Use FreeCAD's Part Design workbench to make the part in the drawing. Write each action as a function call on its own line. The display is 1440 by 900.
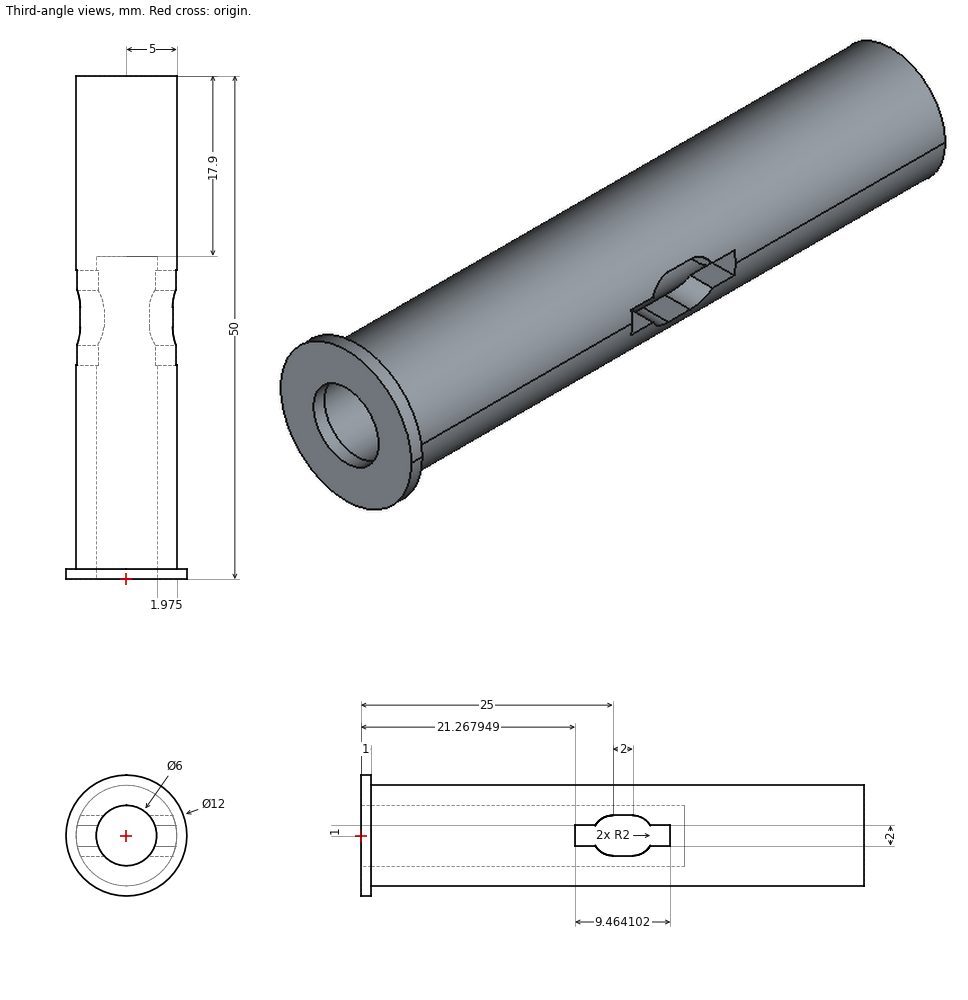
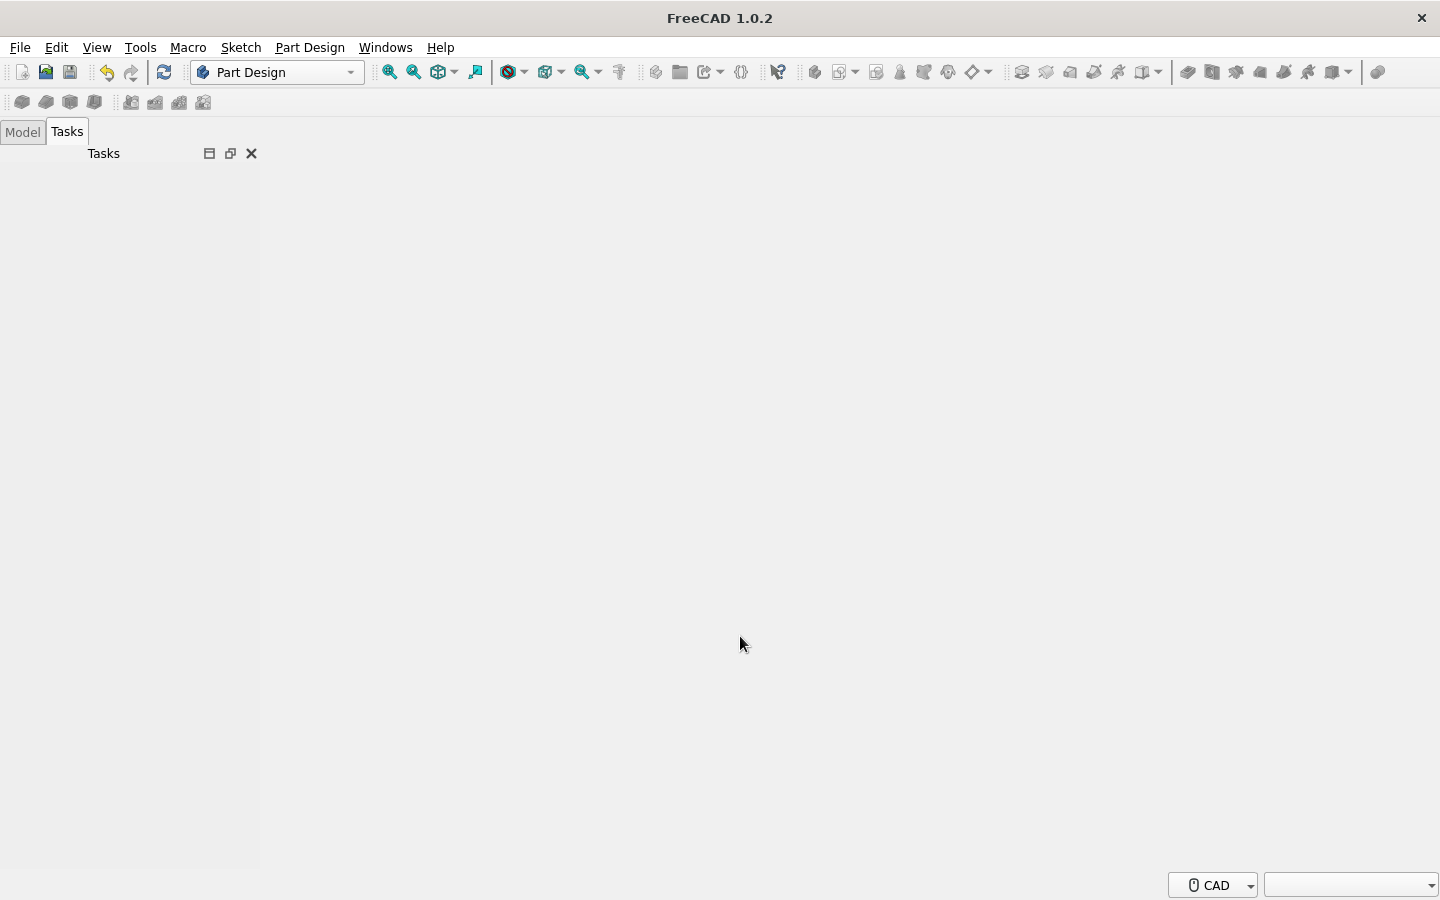
key(ctrl+n)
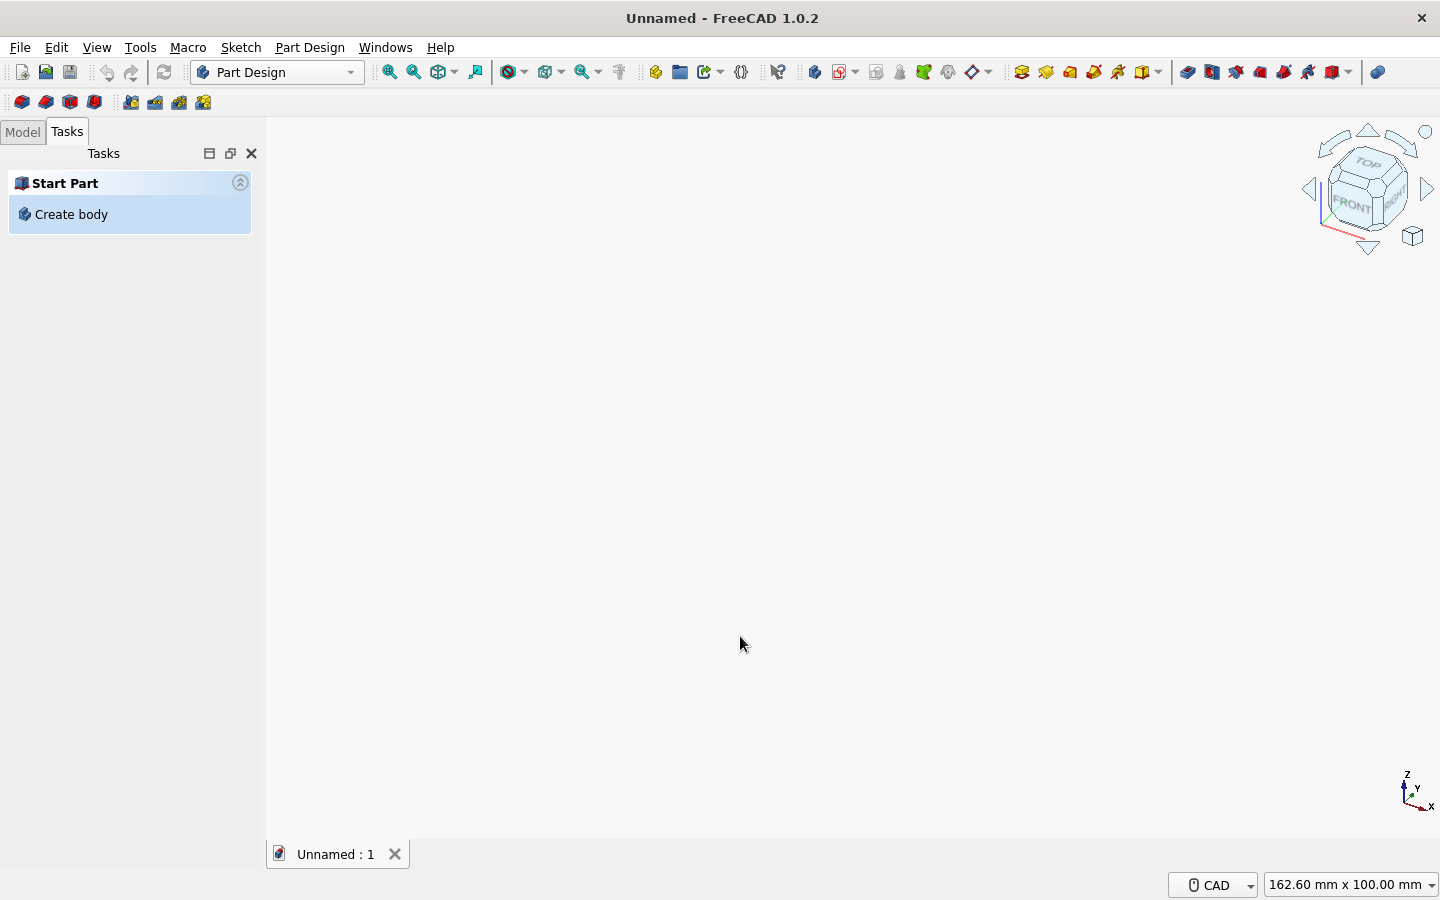
click(840, 72)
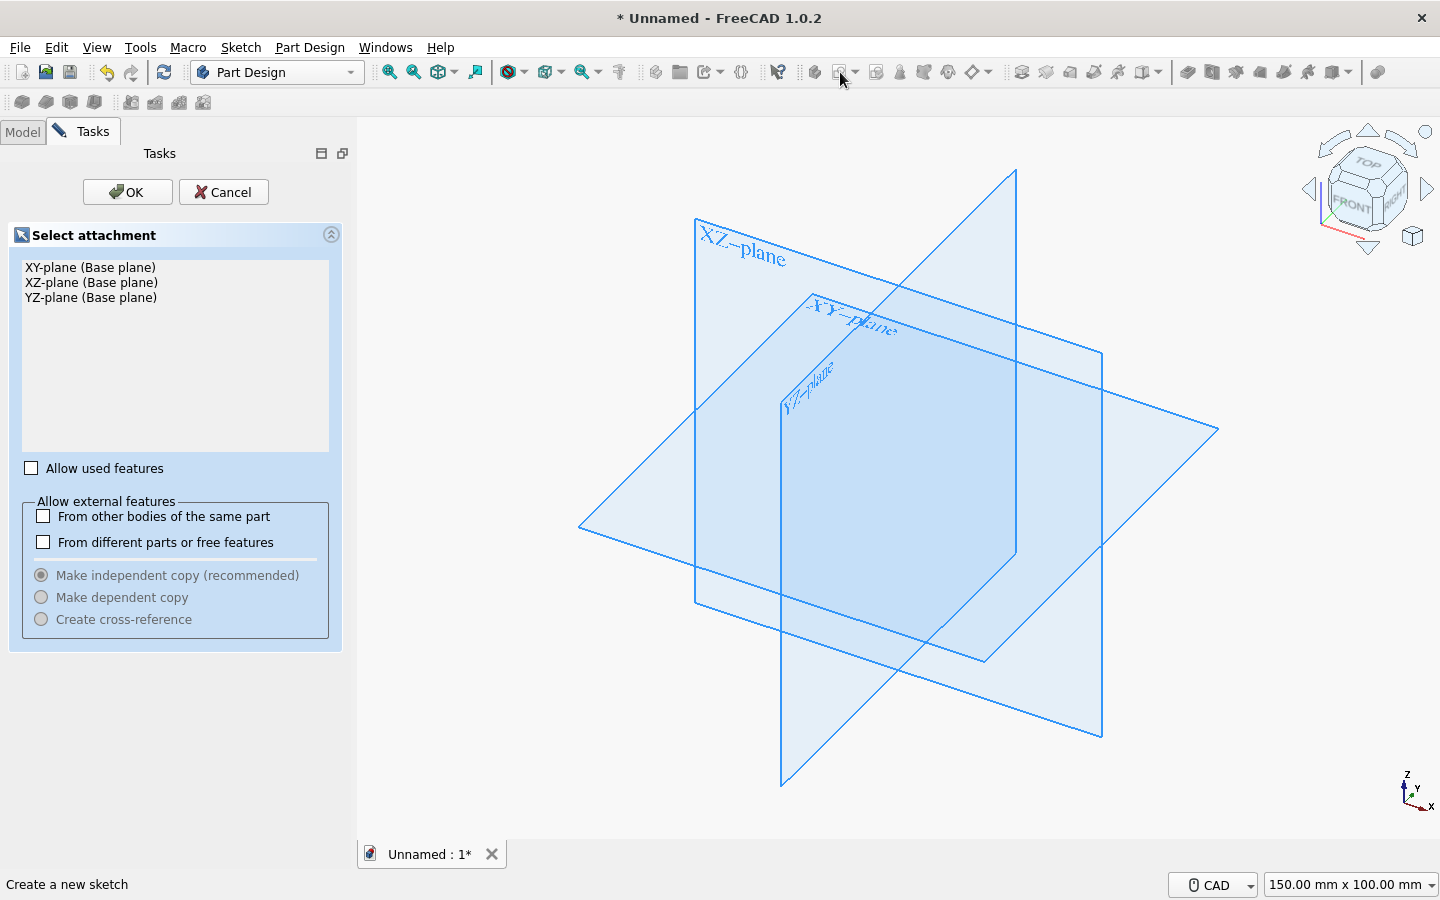
click(82, 268)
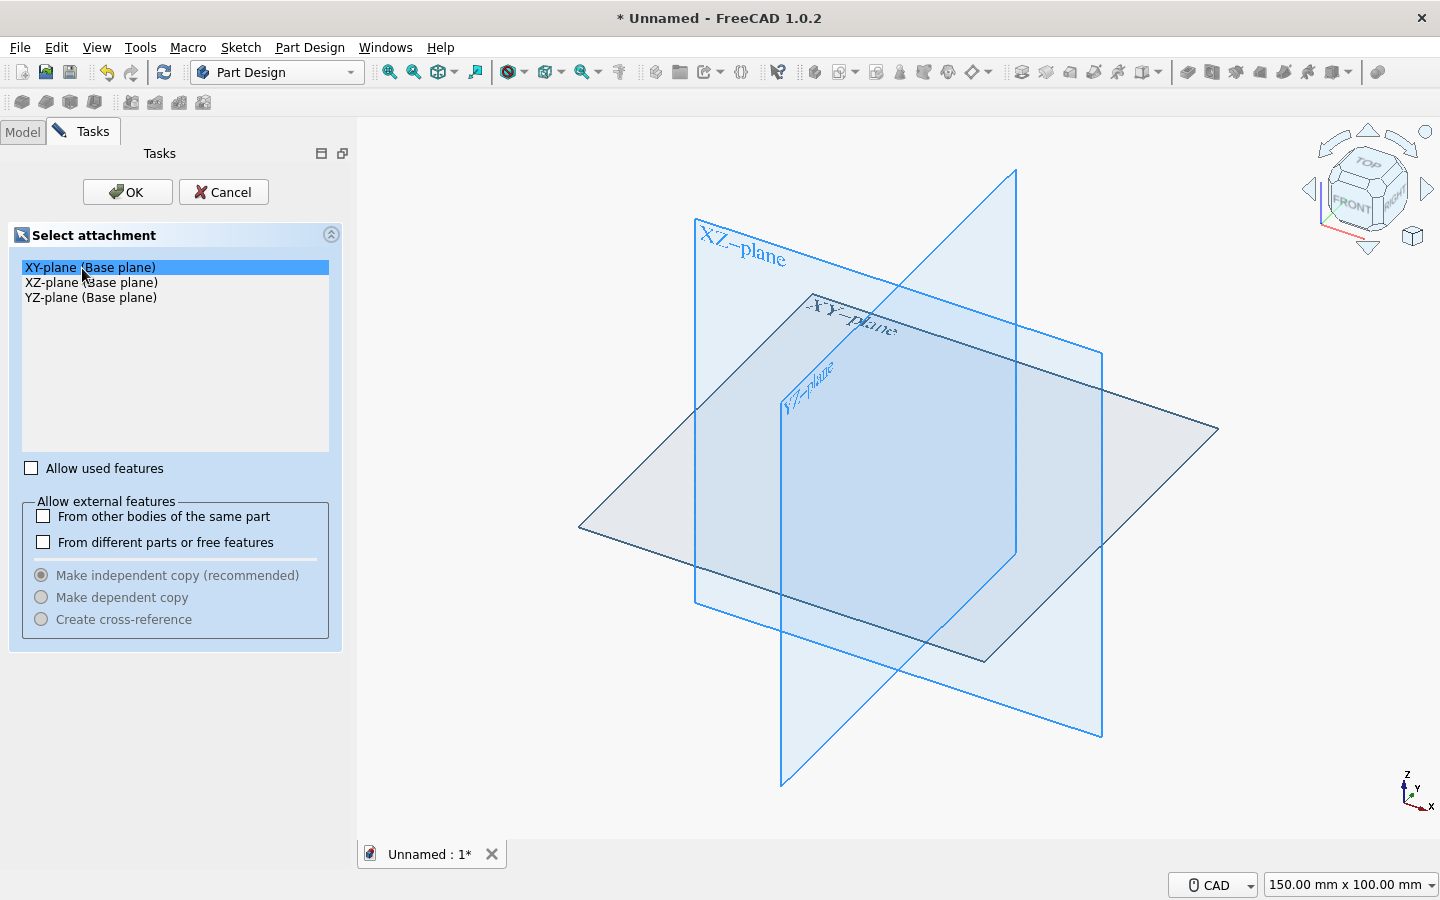
click(128, 192)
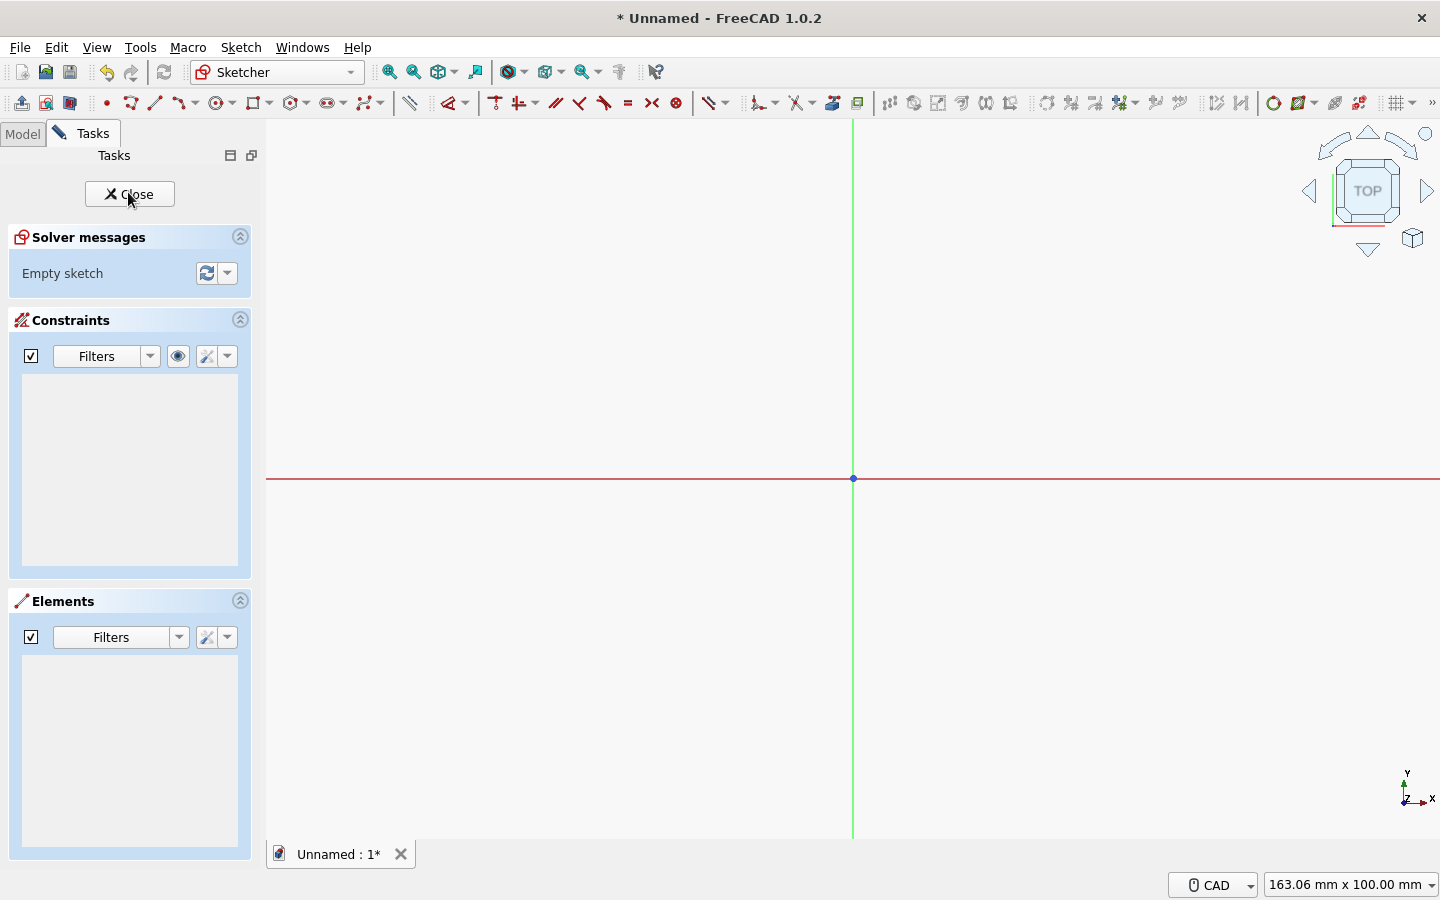
scroll(394, 811, down, 1)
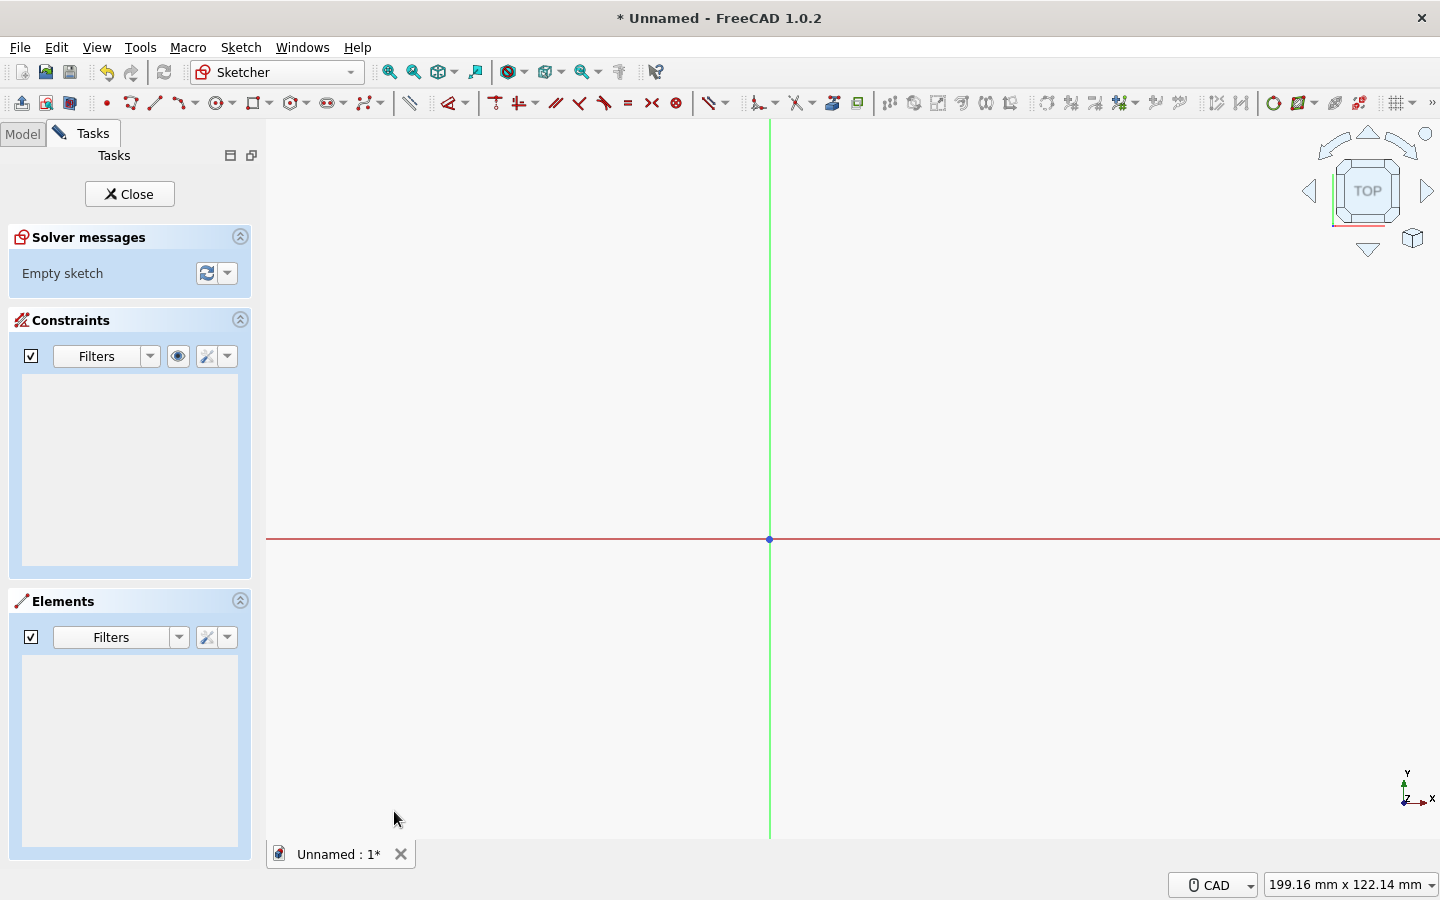
scroll(785, 215, up, 2)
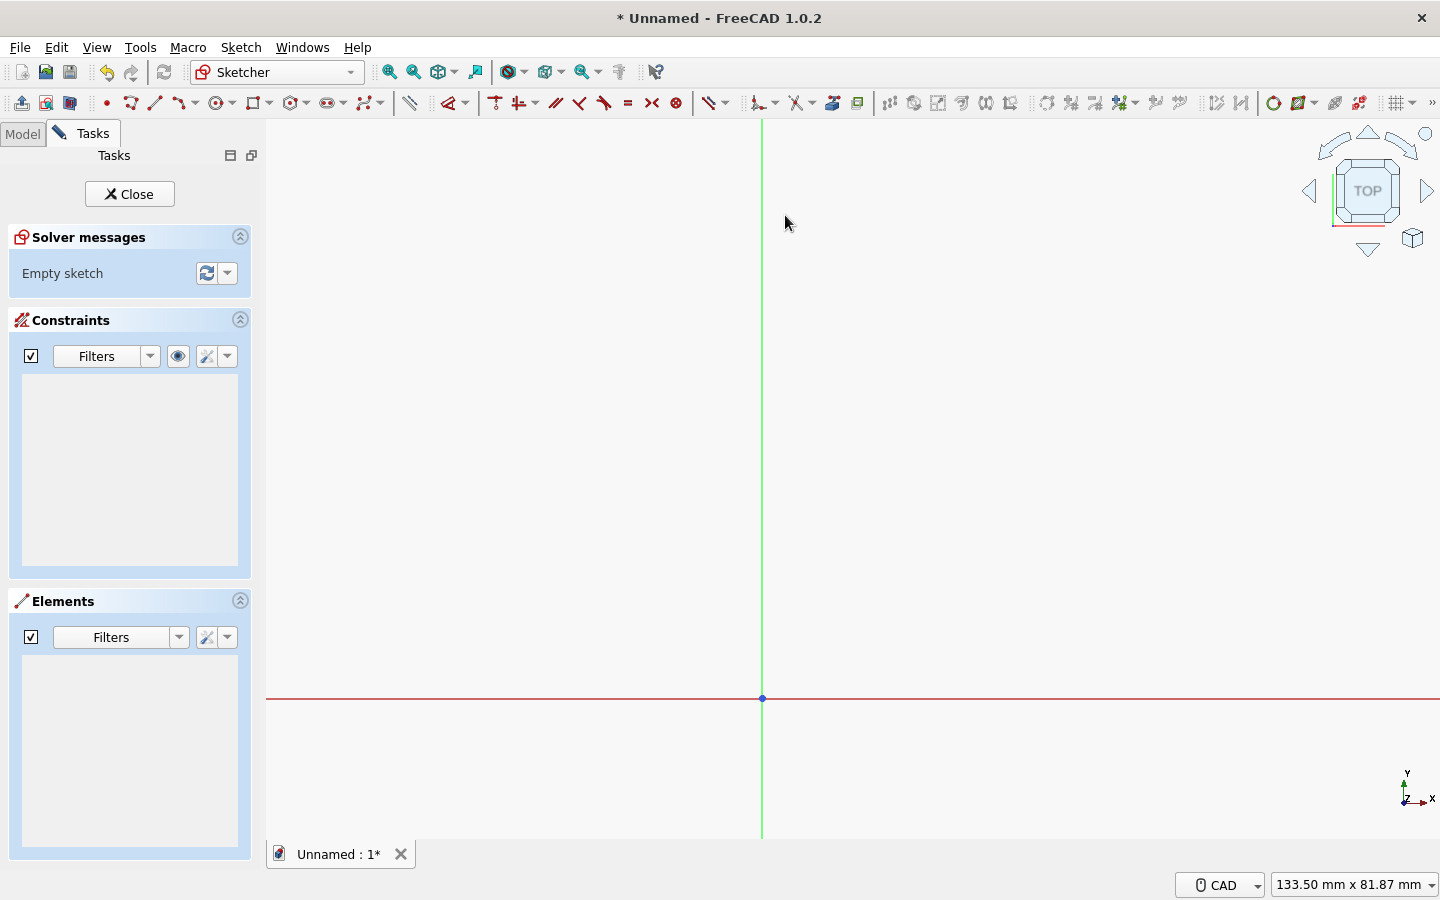
click(132, 104)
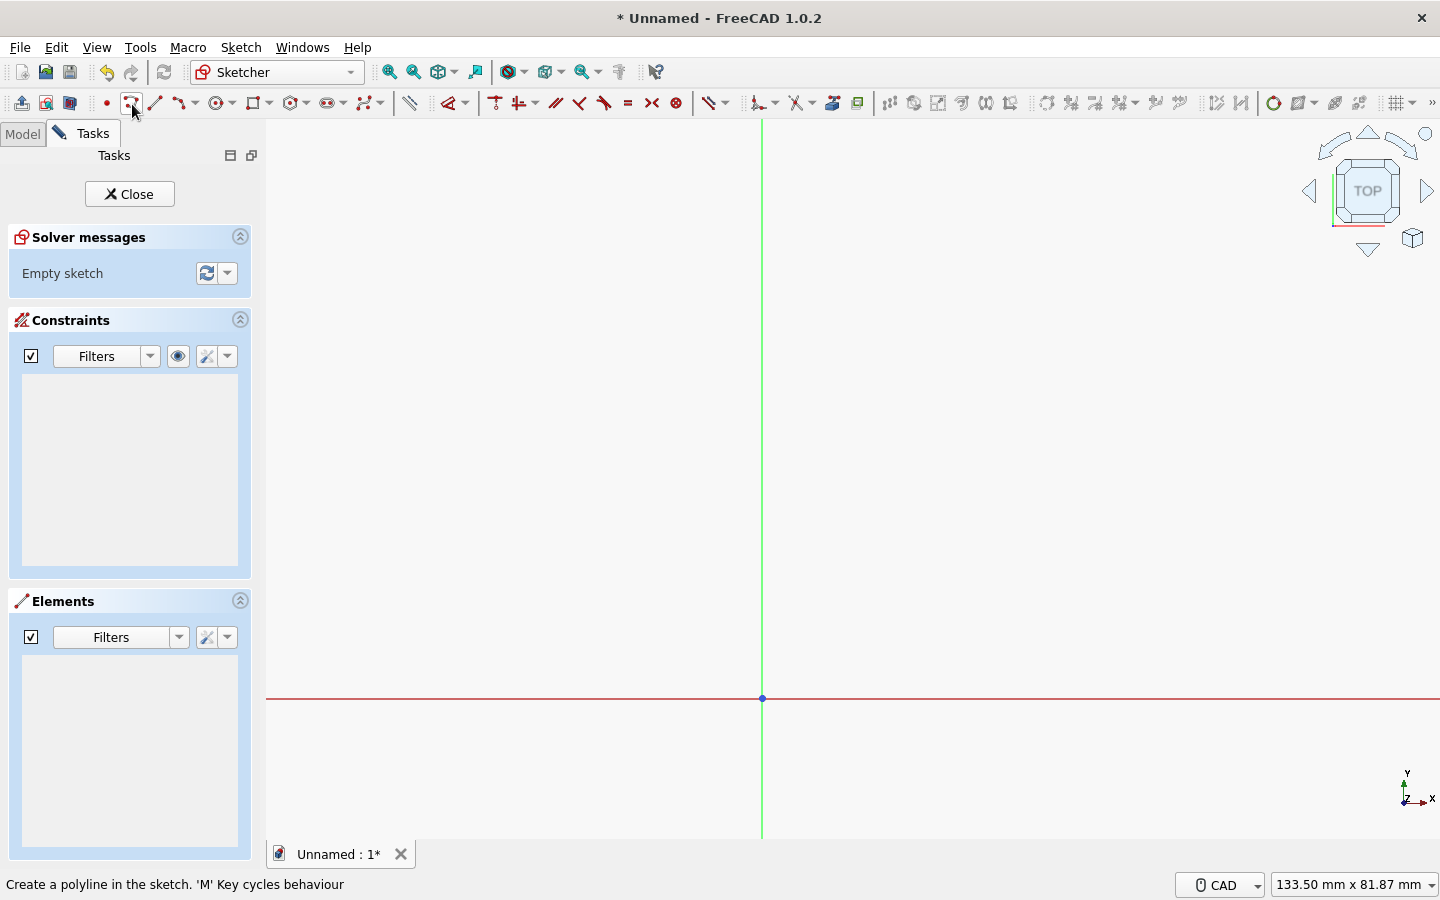
click(789, 699)
click(806, 690)
click(806, 259)
click(762, 259)
click(771, 417)
click(789, 417)